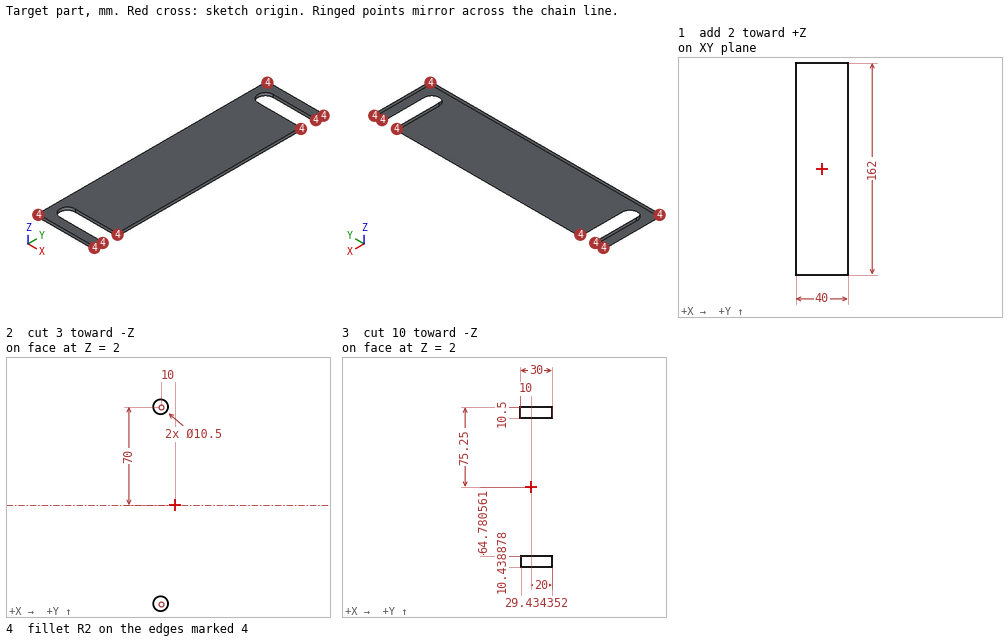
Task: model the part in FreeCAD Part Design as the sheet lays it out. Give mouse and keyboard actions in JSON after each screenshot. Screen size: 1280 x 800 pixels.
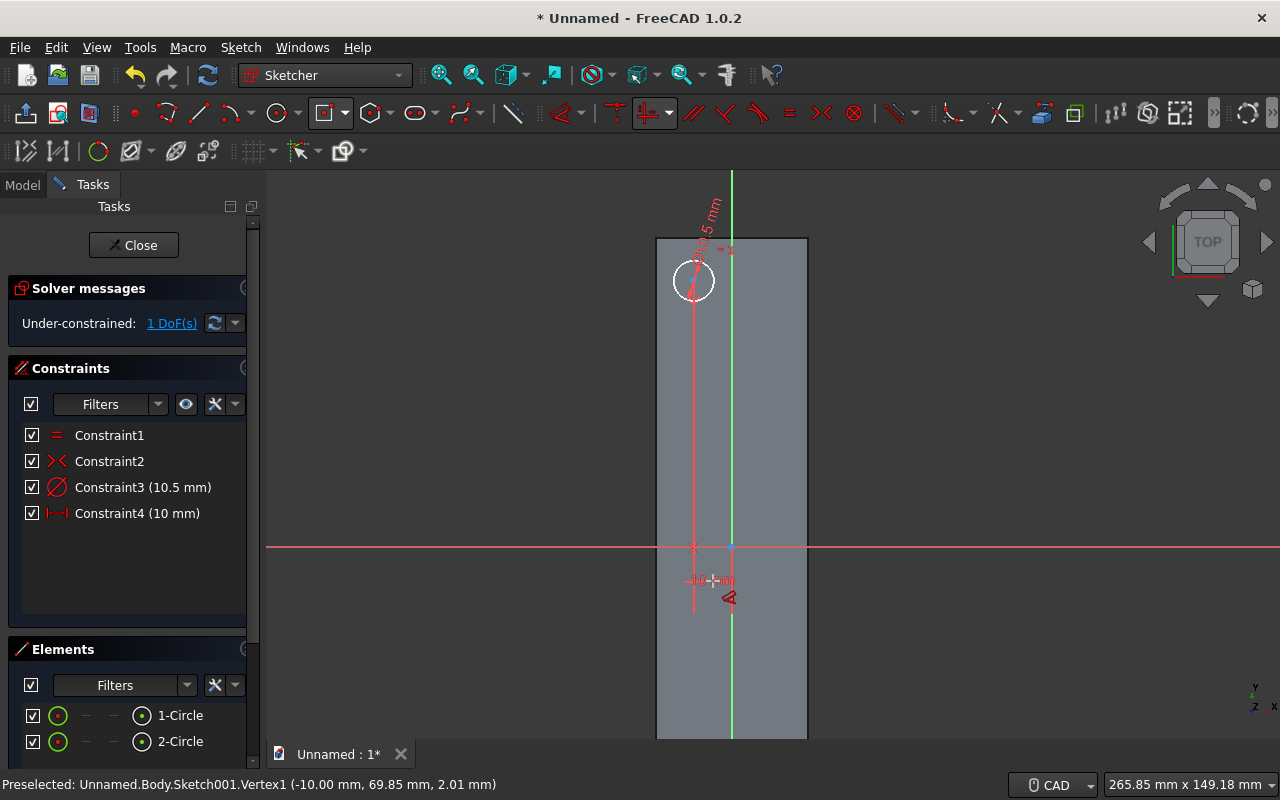
{"action": "left_click", "coordinate": [694, 281]}
{"action": "left_click", "coordinate": [766, 414]}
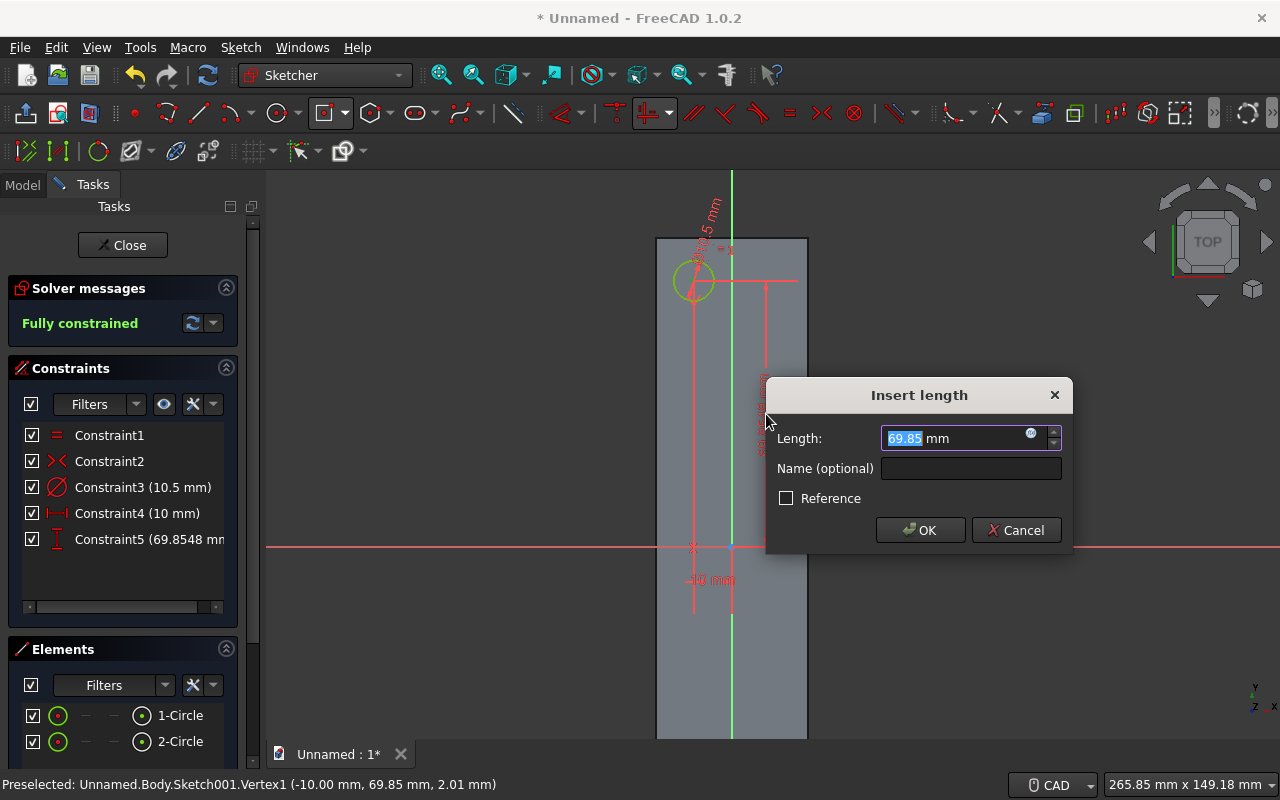
{"action": "type", "text": "70"}
{"action": "key", "text": "Return"}
{"action": "key", "text": "Escape"}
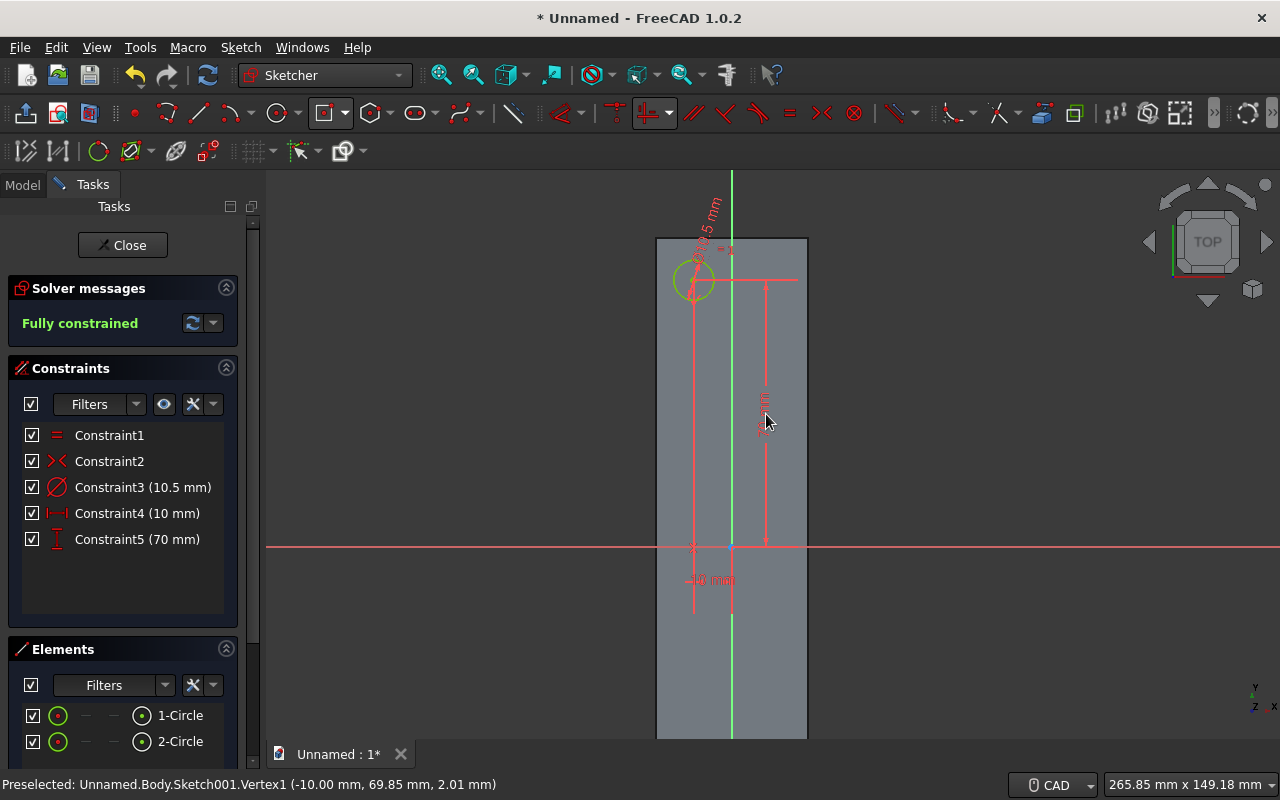
{"action": "left_click", "coordinate": [123, 245]}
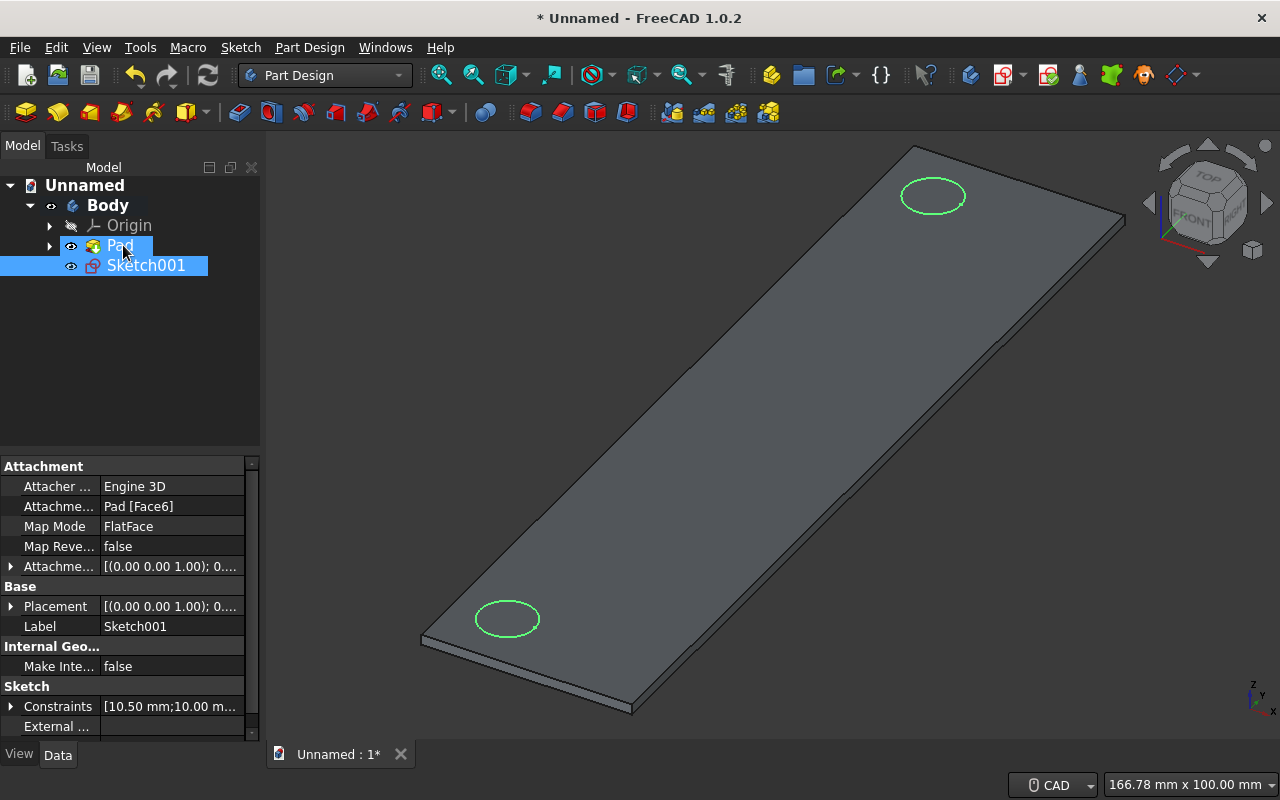
{"action": "left_click", "coordinate": [240, 112]}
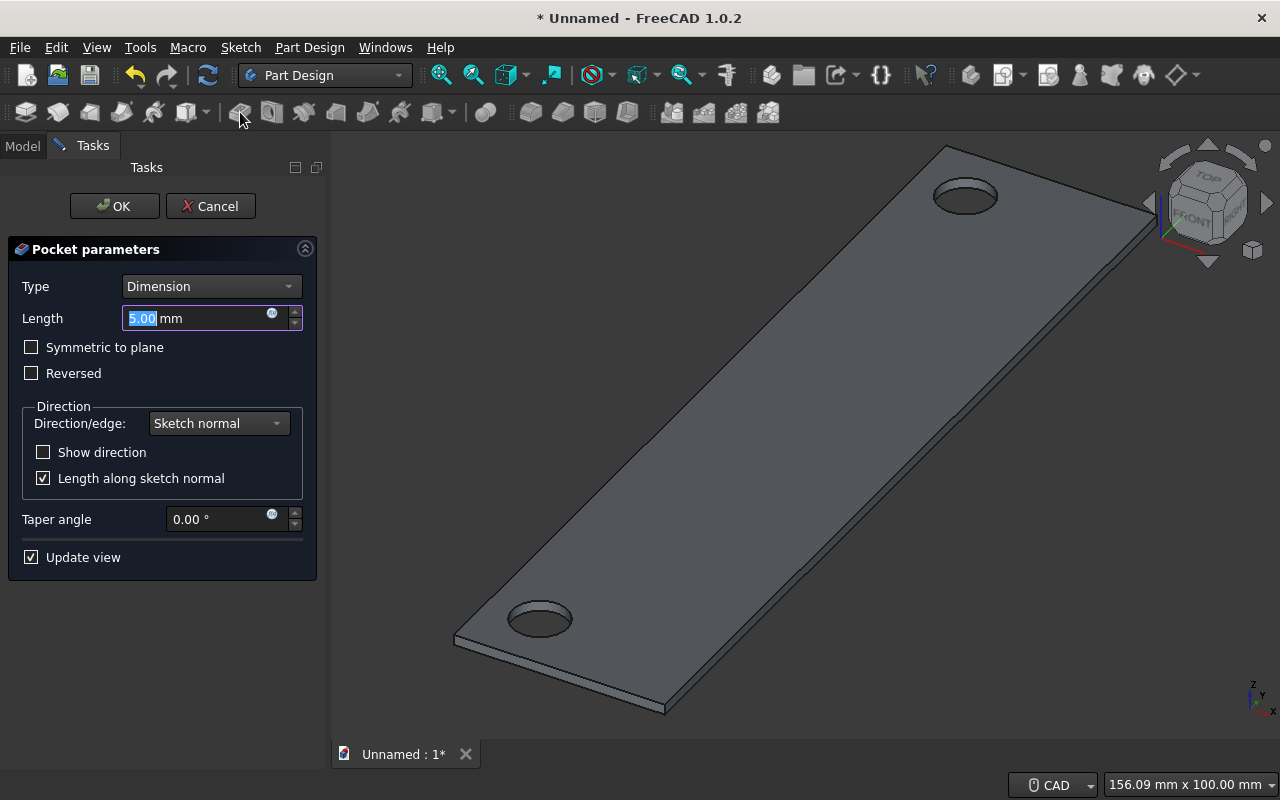
{"action": "type", "text": "3"}
{"action": "key", "text": "Tab"}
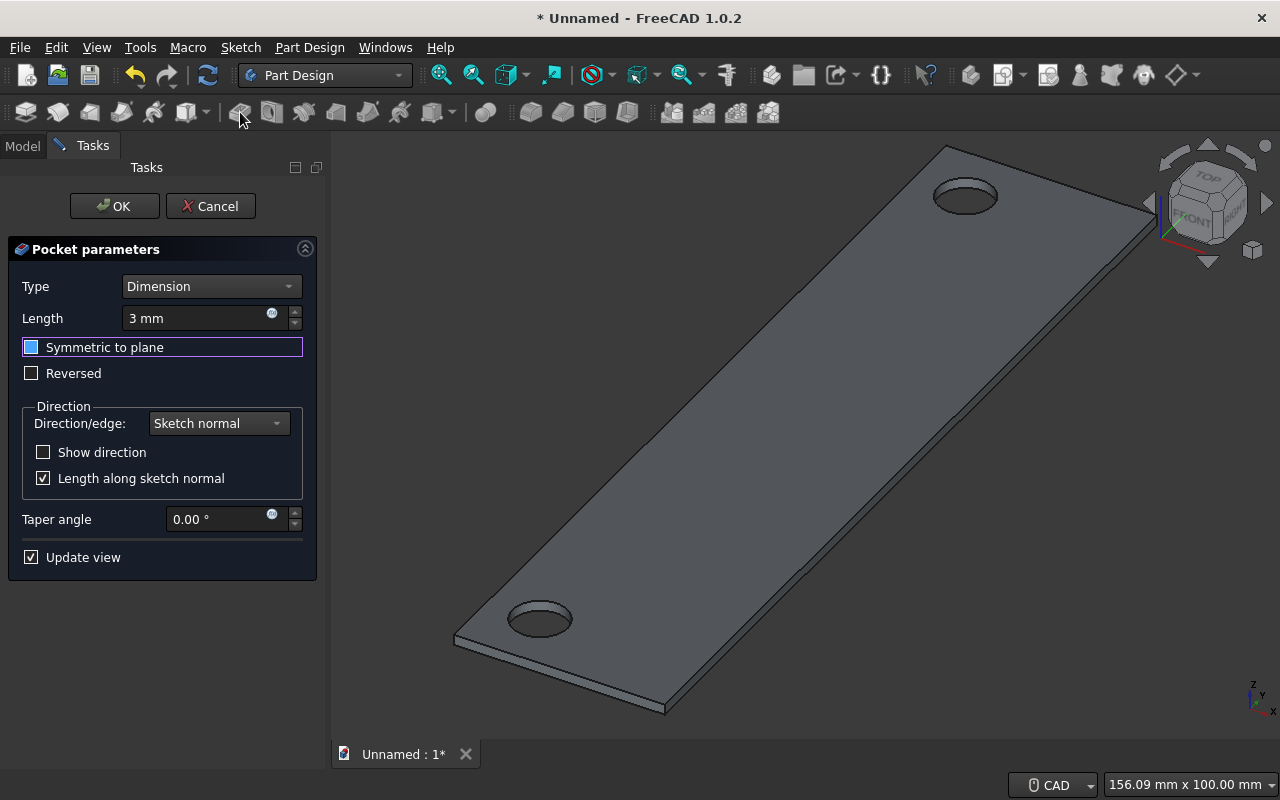
{"action": "left_click", "coordinate": [115, 206]}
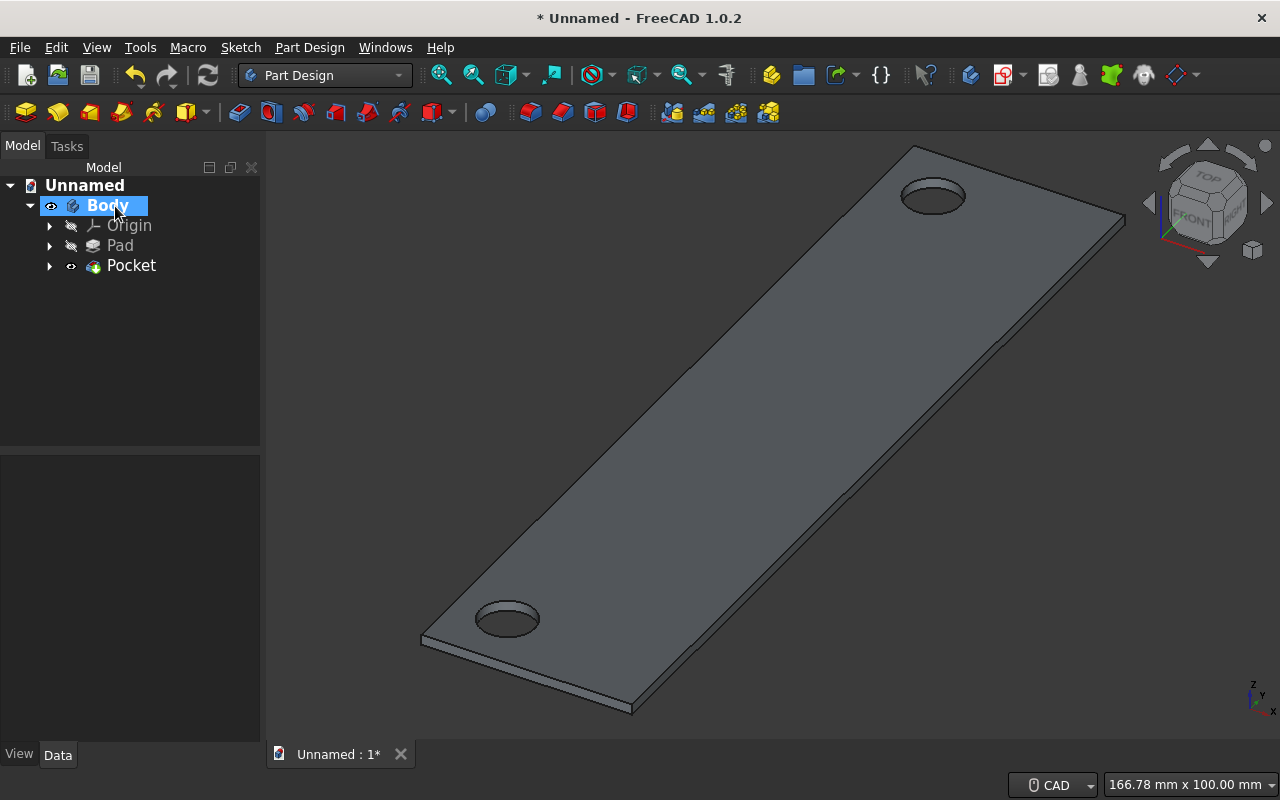
{"action": "left_click", "coordinate": [914, 284]}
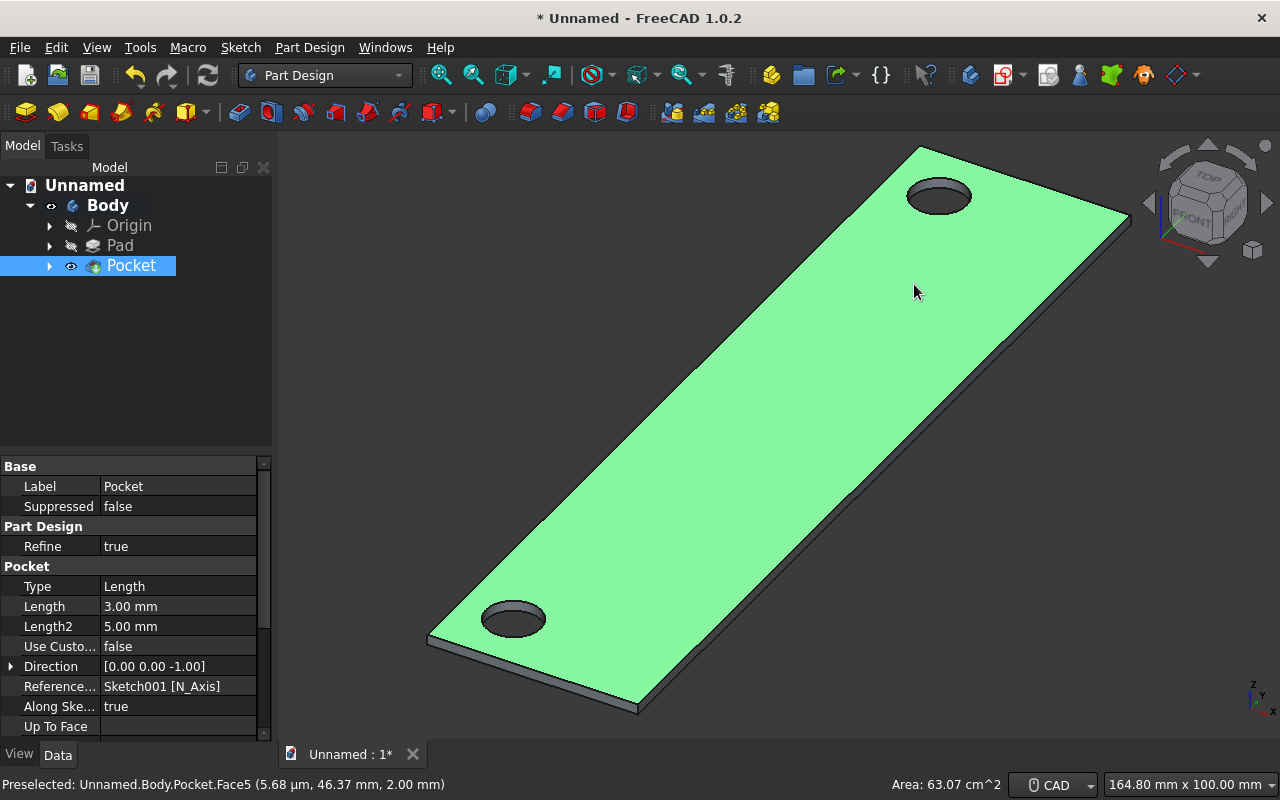
{"action": "left_click", "coordinate": [1004, 76]}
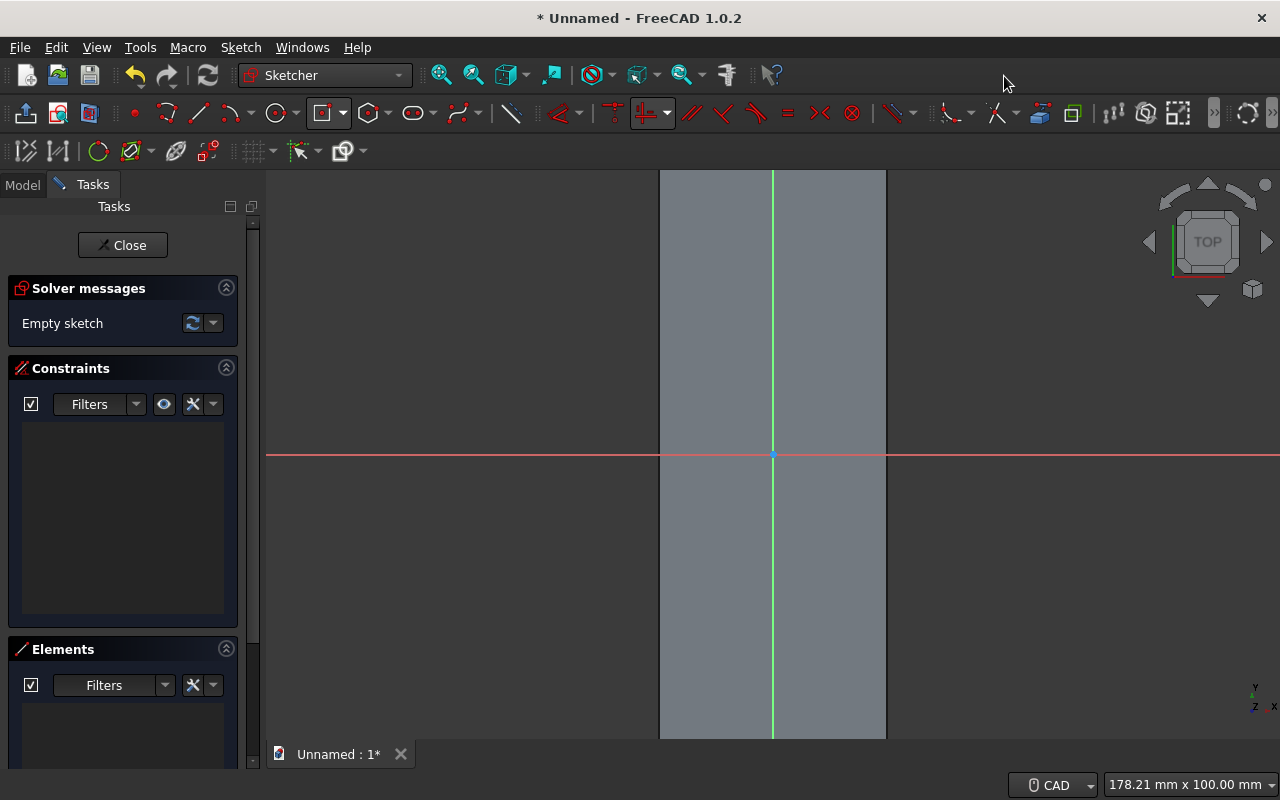
{"action": "scroll", "coordinate": [625, 455], "scroll_direction": "down", "scroll_amount": 4}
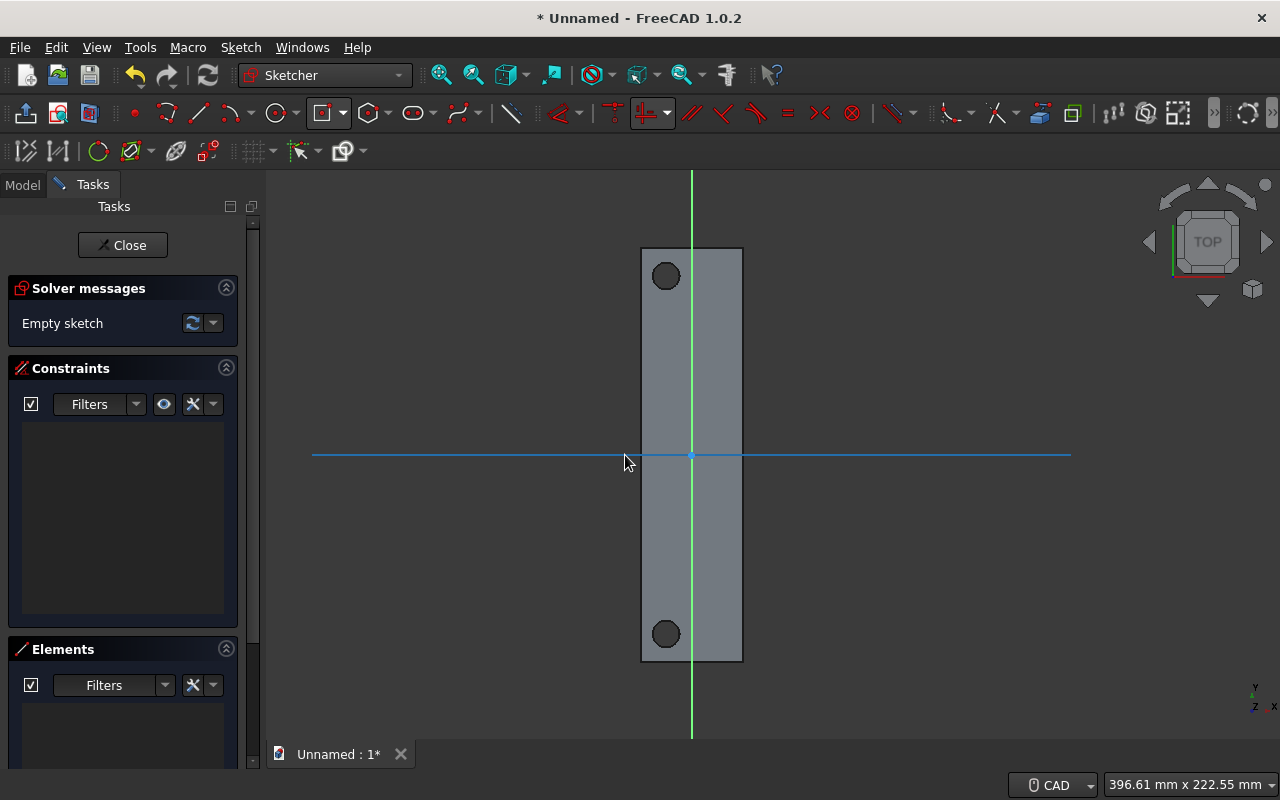
{"action": "key", "text": "g r"}